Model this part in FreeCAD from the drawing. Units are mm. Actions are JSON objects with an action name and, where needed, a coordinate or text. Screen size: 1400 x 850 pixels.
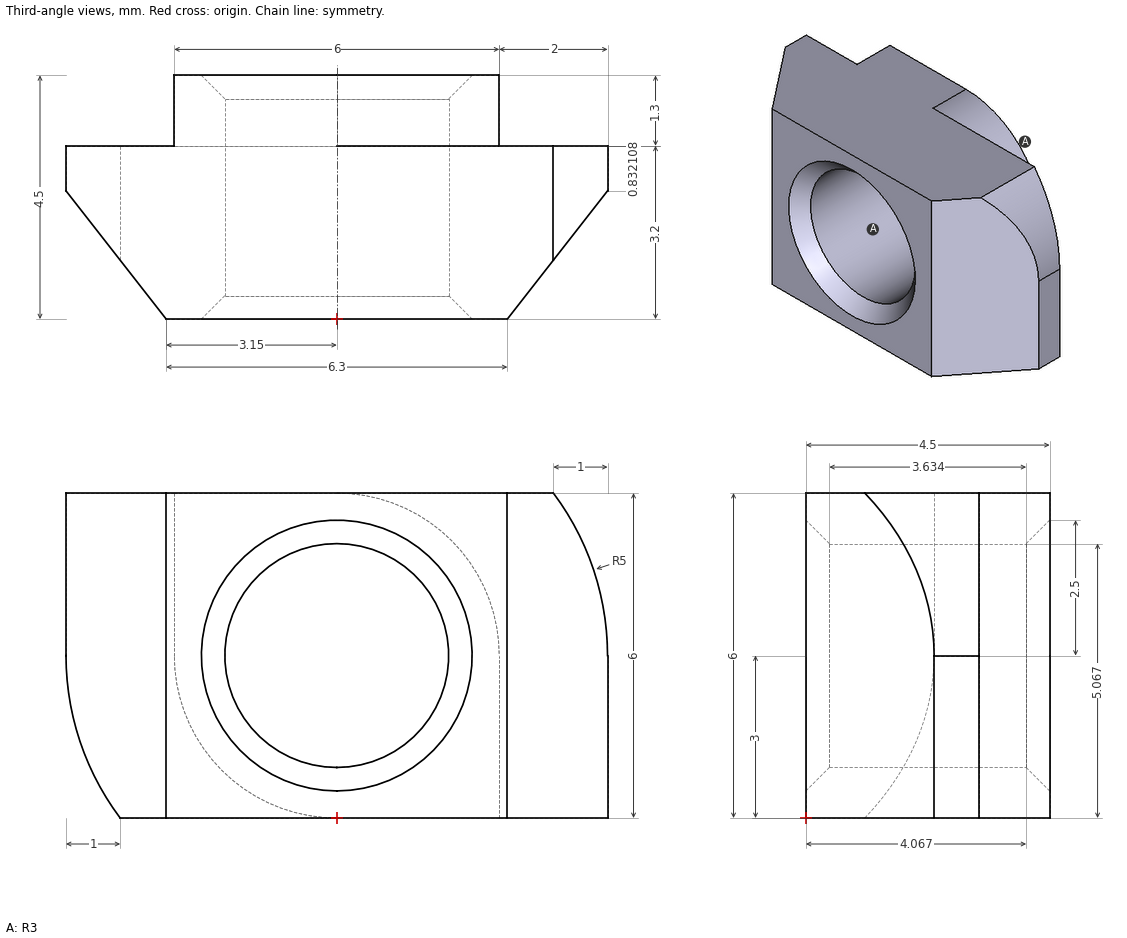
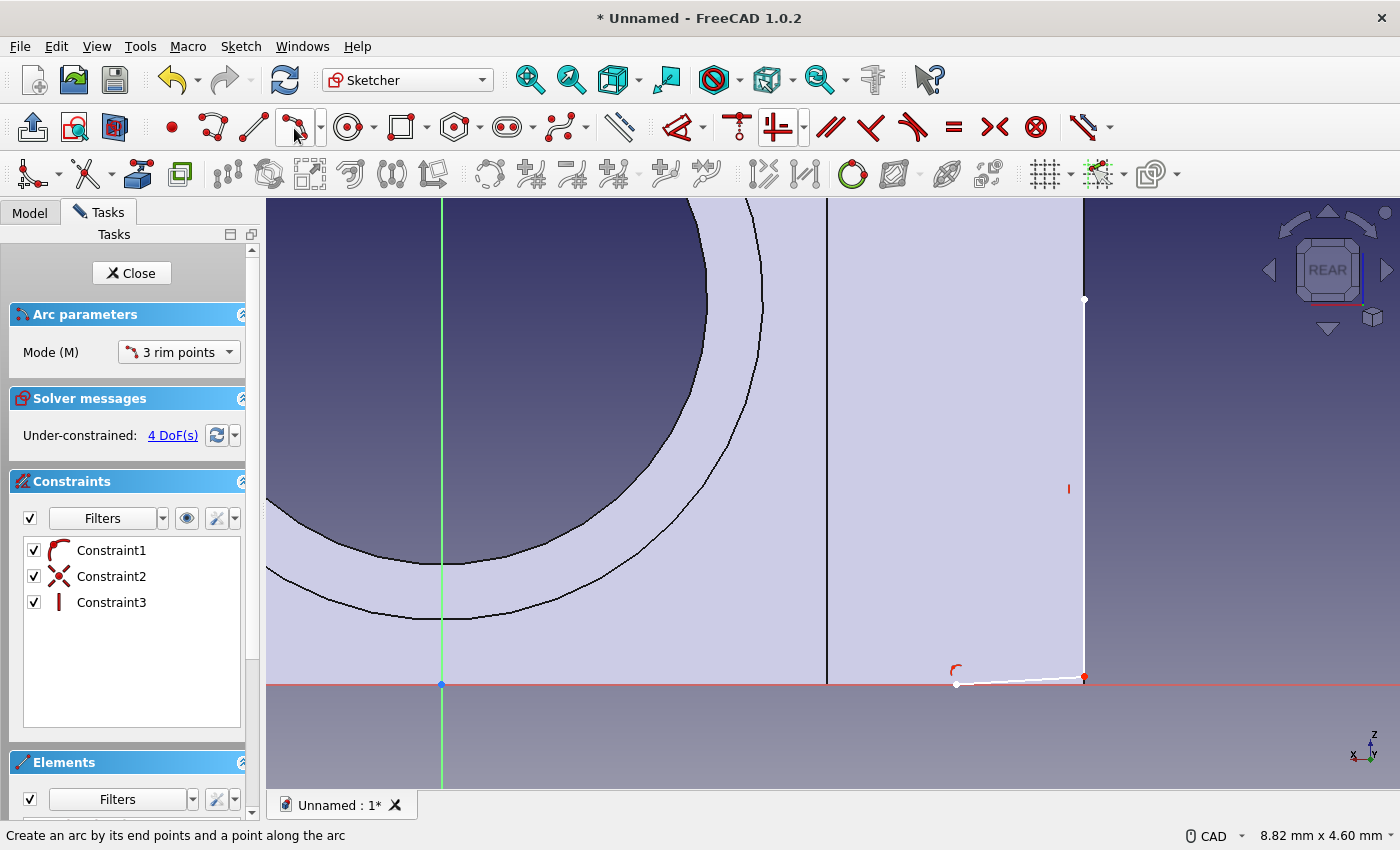
{"action": "left_click", "coordinate": [1084, 300]}
{"action": "left_click", "coordinate": [956, 685]}
{"action": "left_click", "coordinate": [1051, 502]}
{"action": "key", "text": "Escape"}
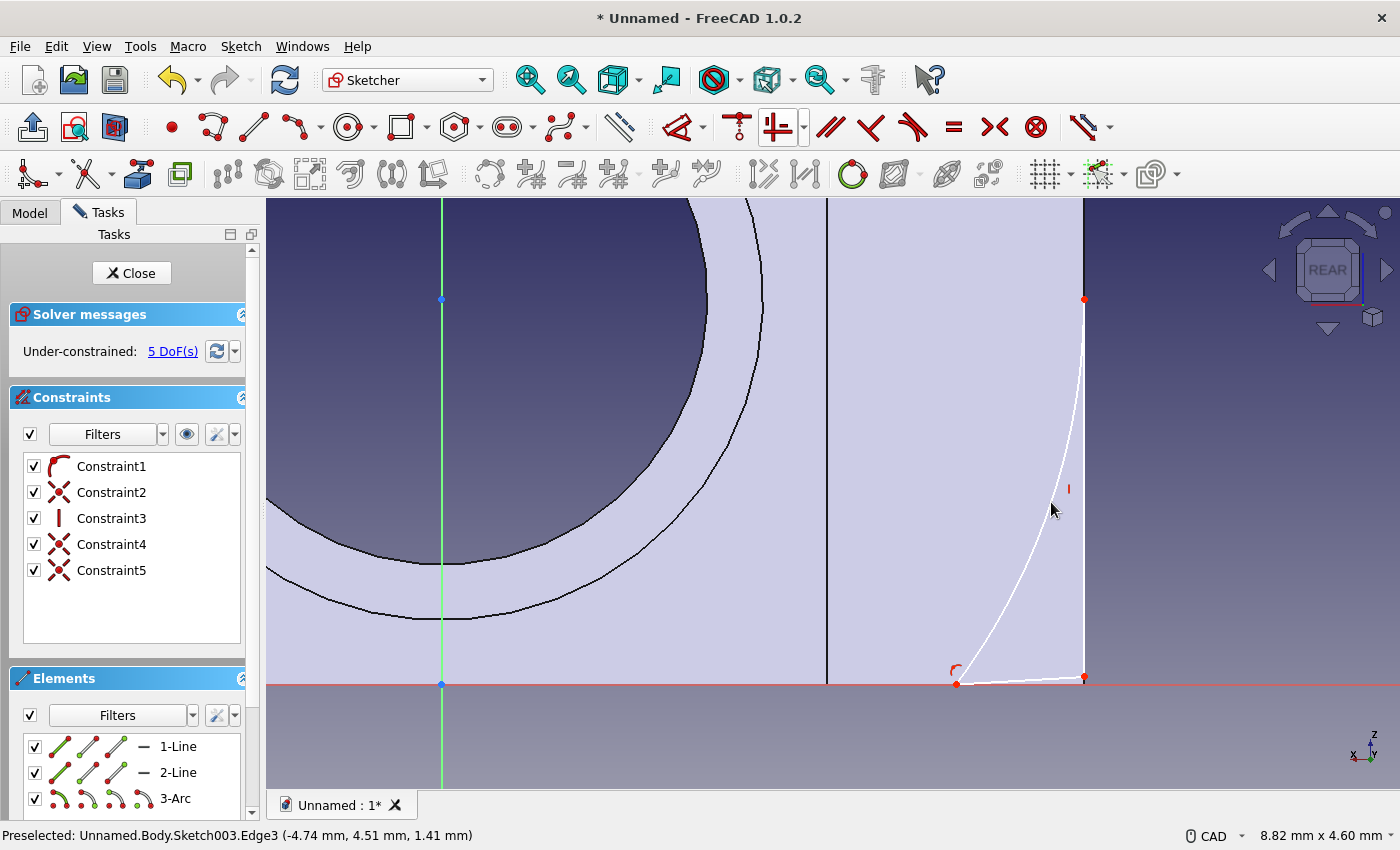
{"action": "left_click", "coordinate": [1084, 564]}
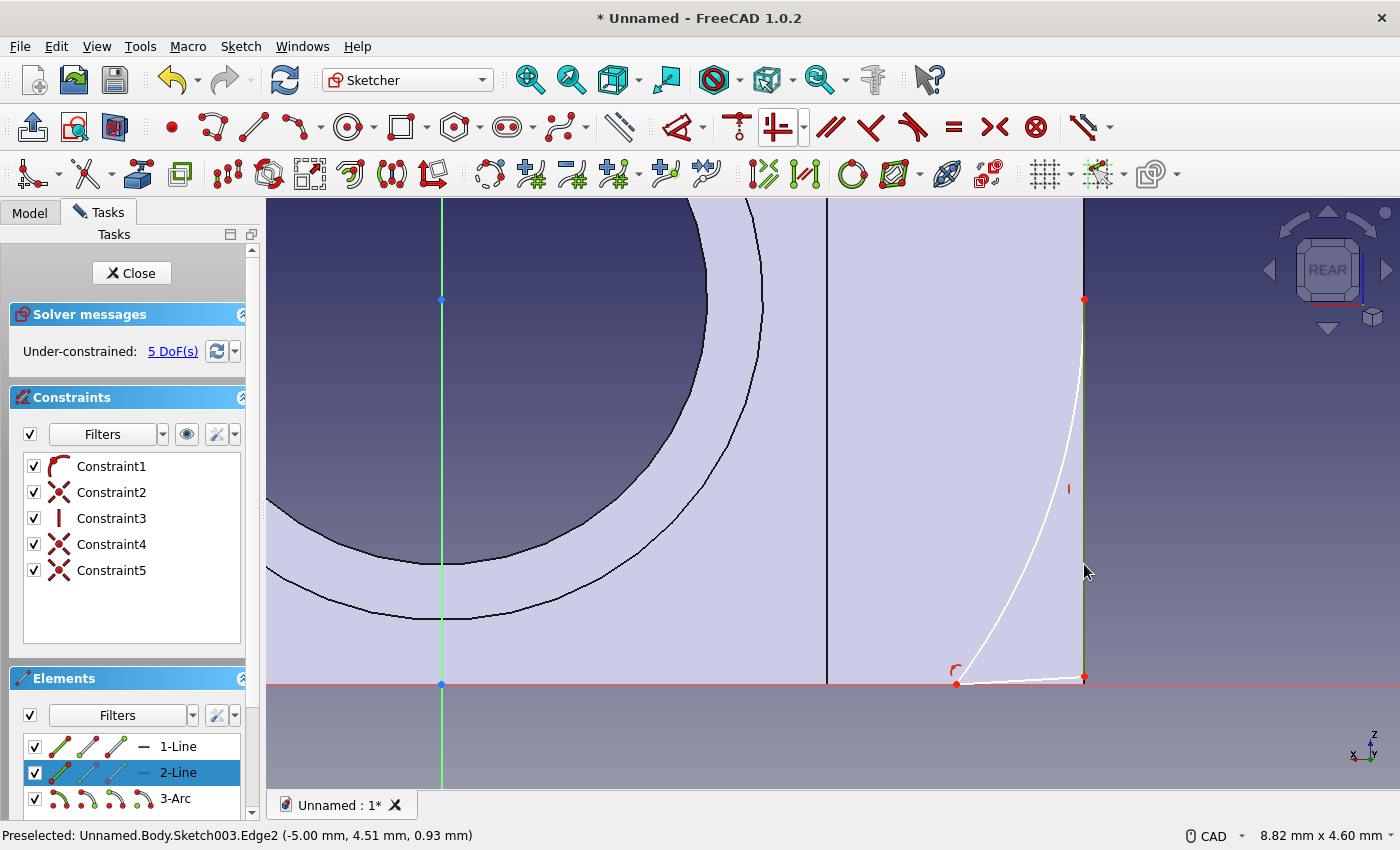
{"action": "left_click", "coordinate": [1020, 579]}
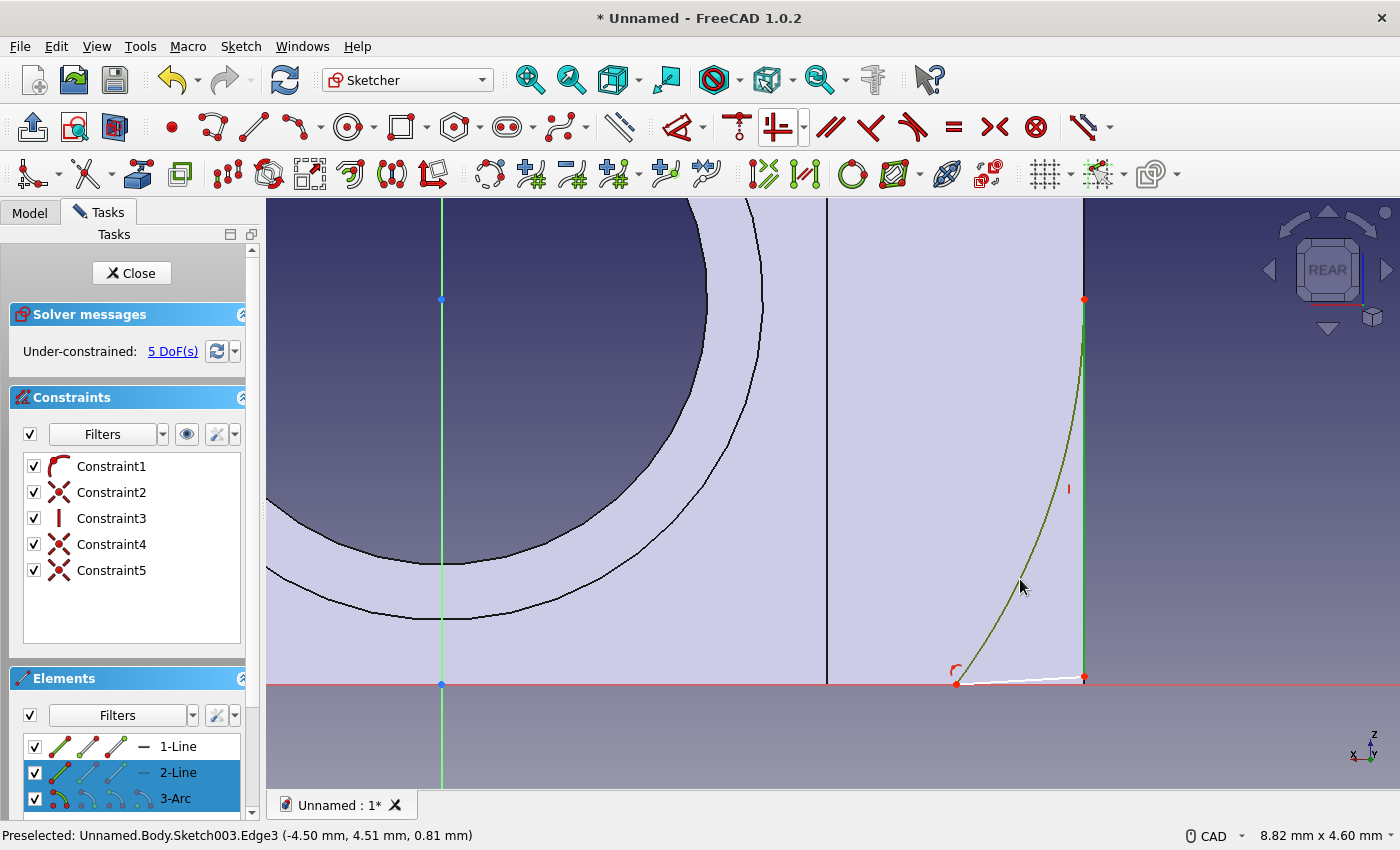
{"action": "left_click", "coordinate": [913, 128]}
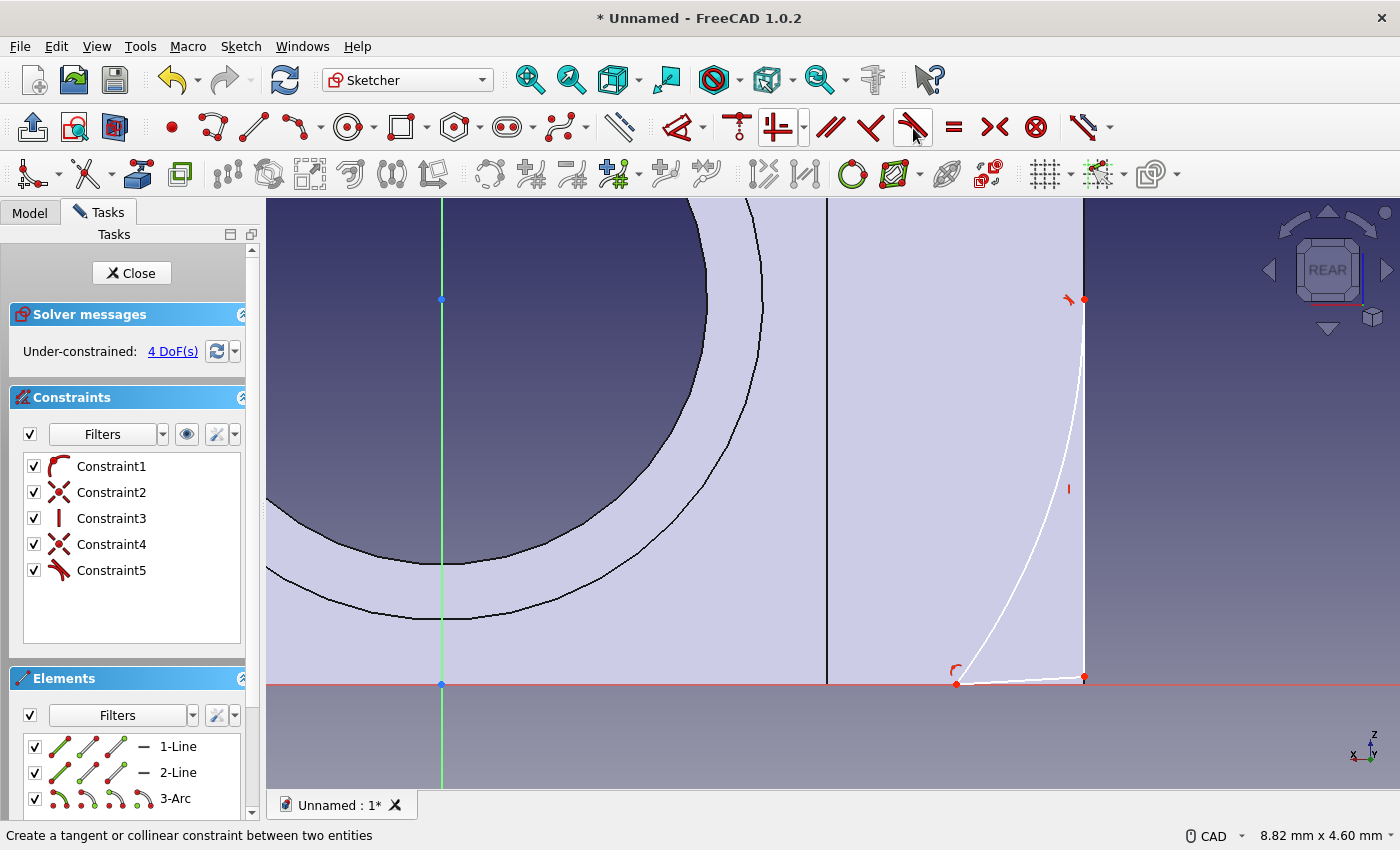
{"action": "left_click", "coordinate": [994, 682]}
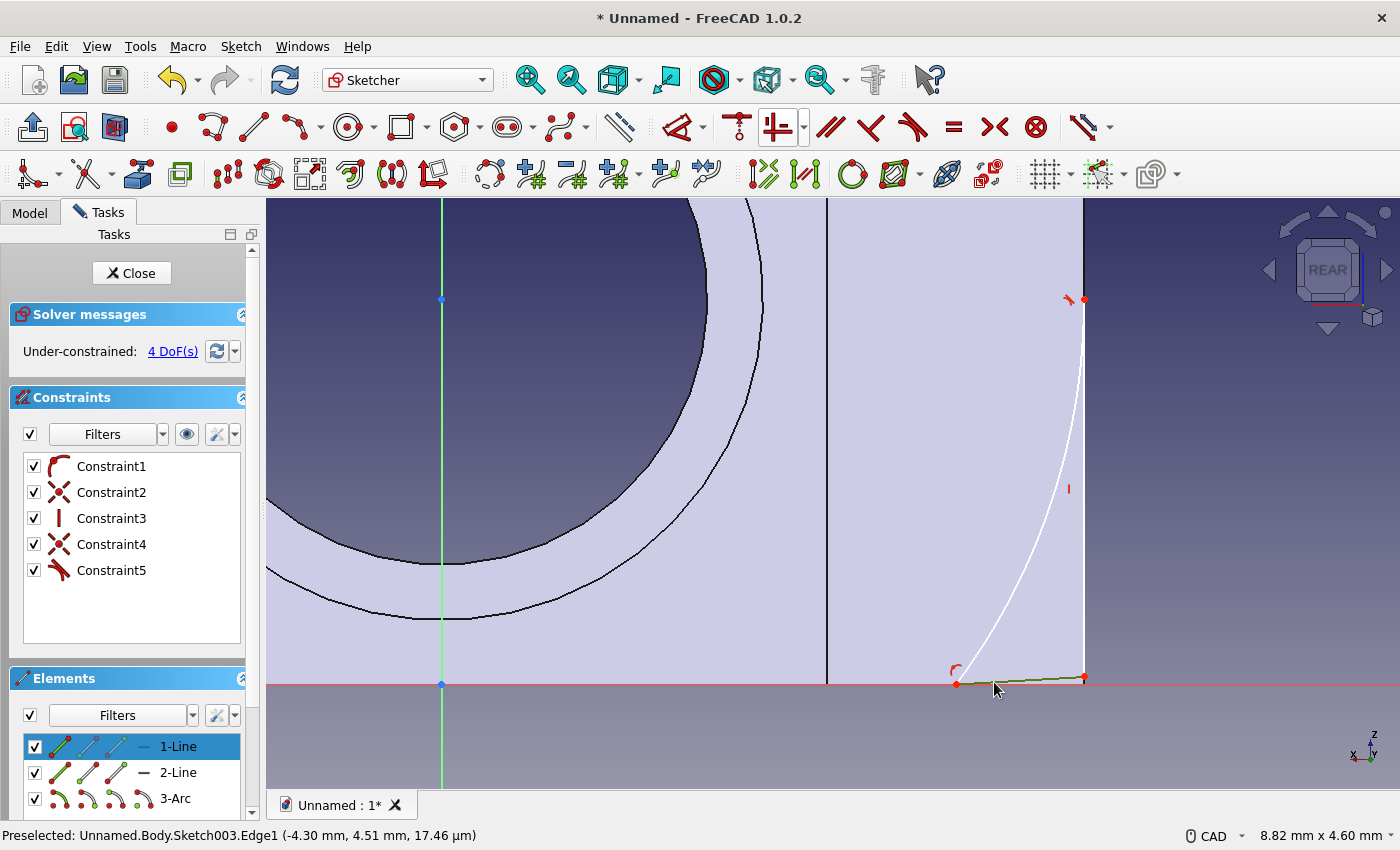
{"action": "left_click", "coordinate": [804, 128]}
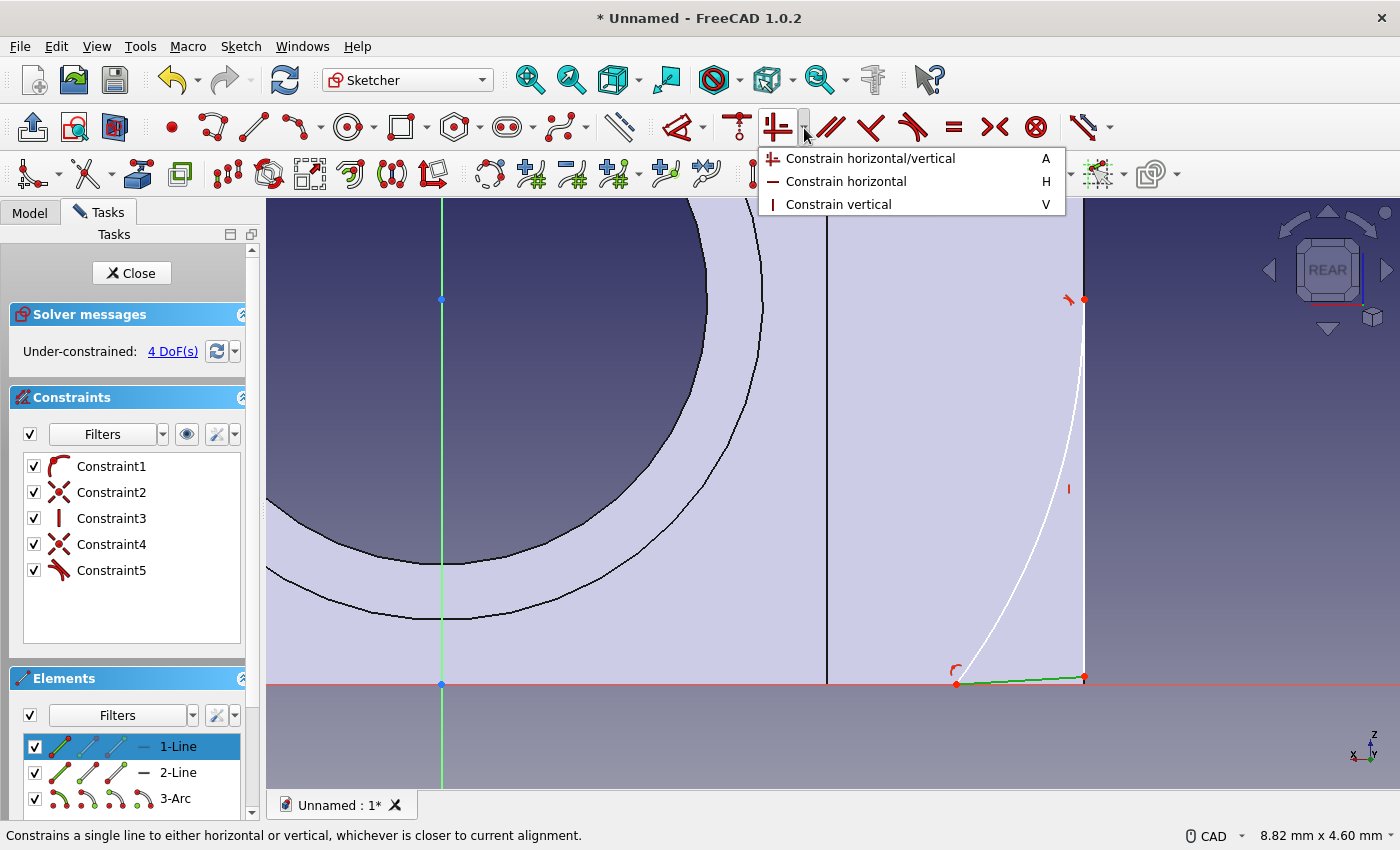
{"action": "left_click", "coordinate": [912, 182]}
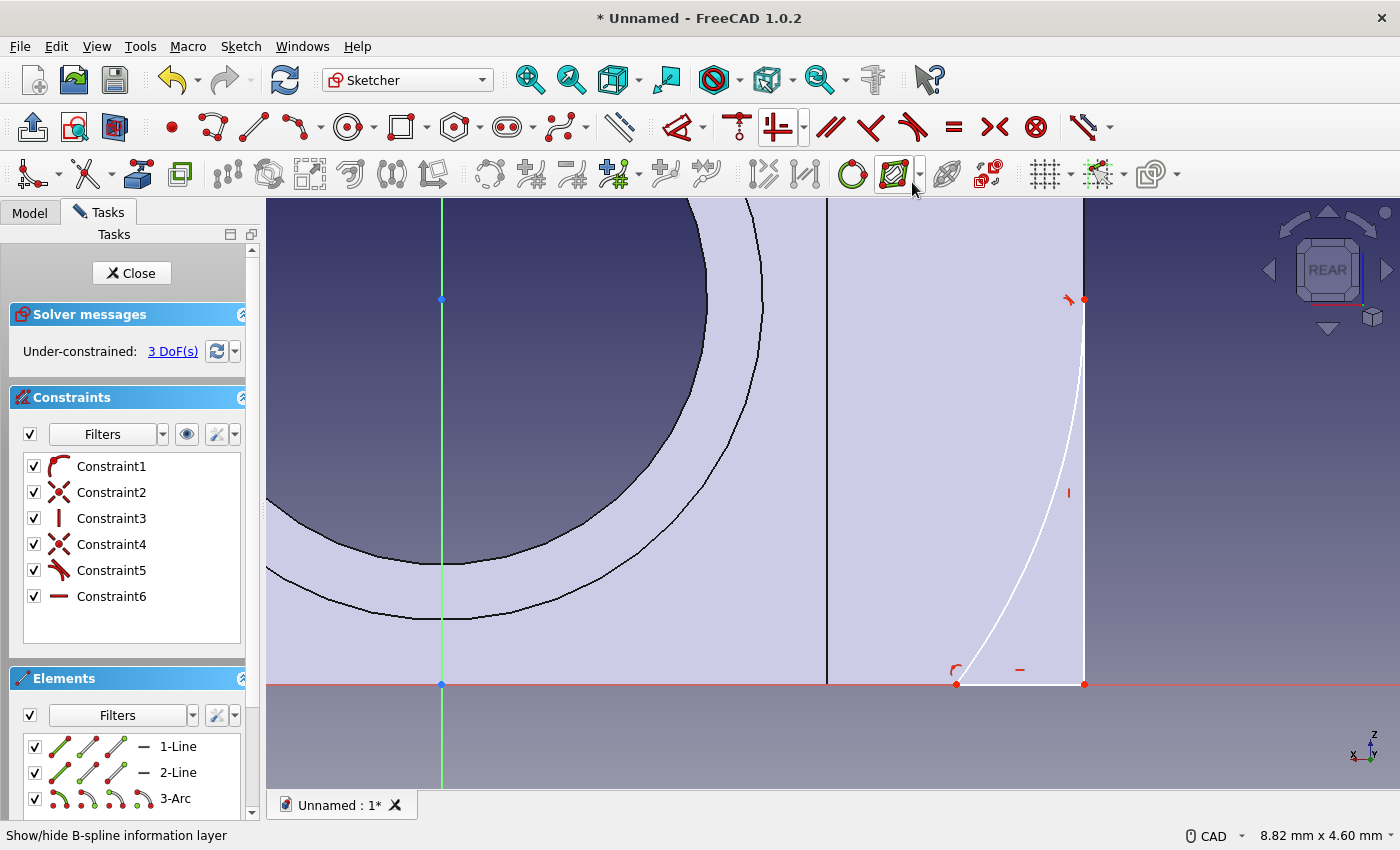
{"action": "left_click", "coordinate": [442, 300]}